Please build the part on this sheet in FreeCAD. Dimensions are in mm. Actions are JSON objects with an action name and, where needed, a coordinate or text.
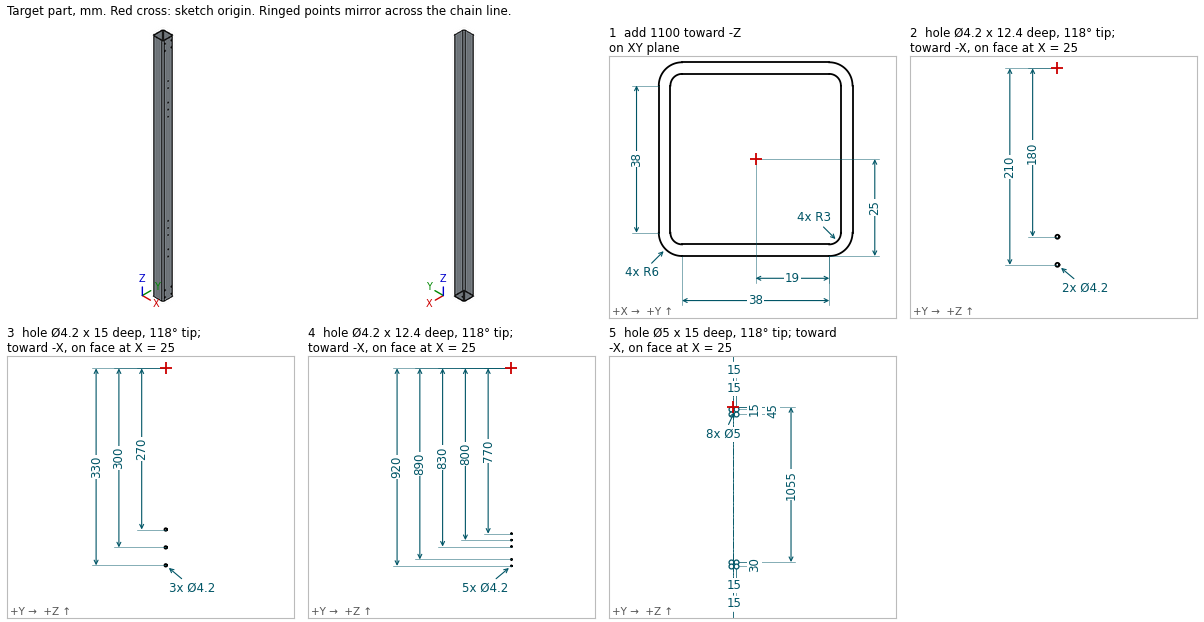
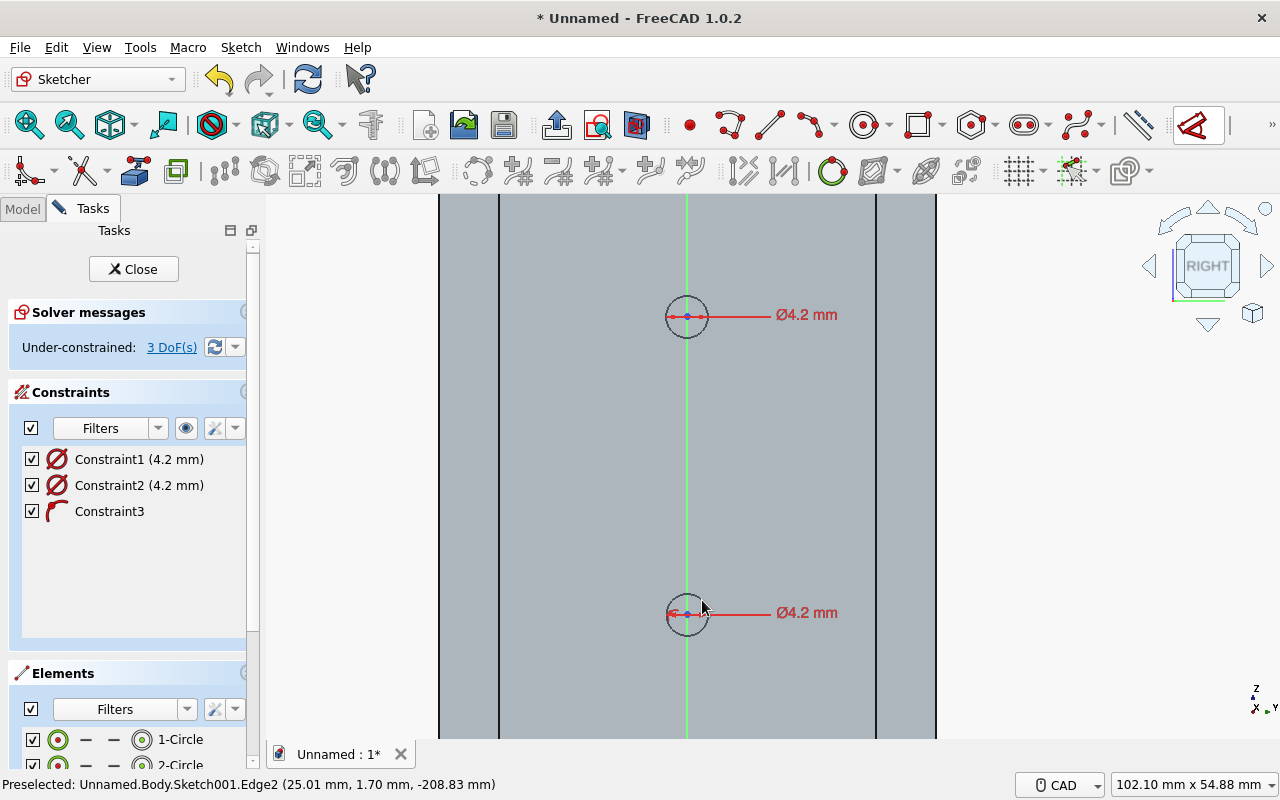
{"action": "left_click", "coordinate": [687, 317]}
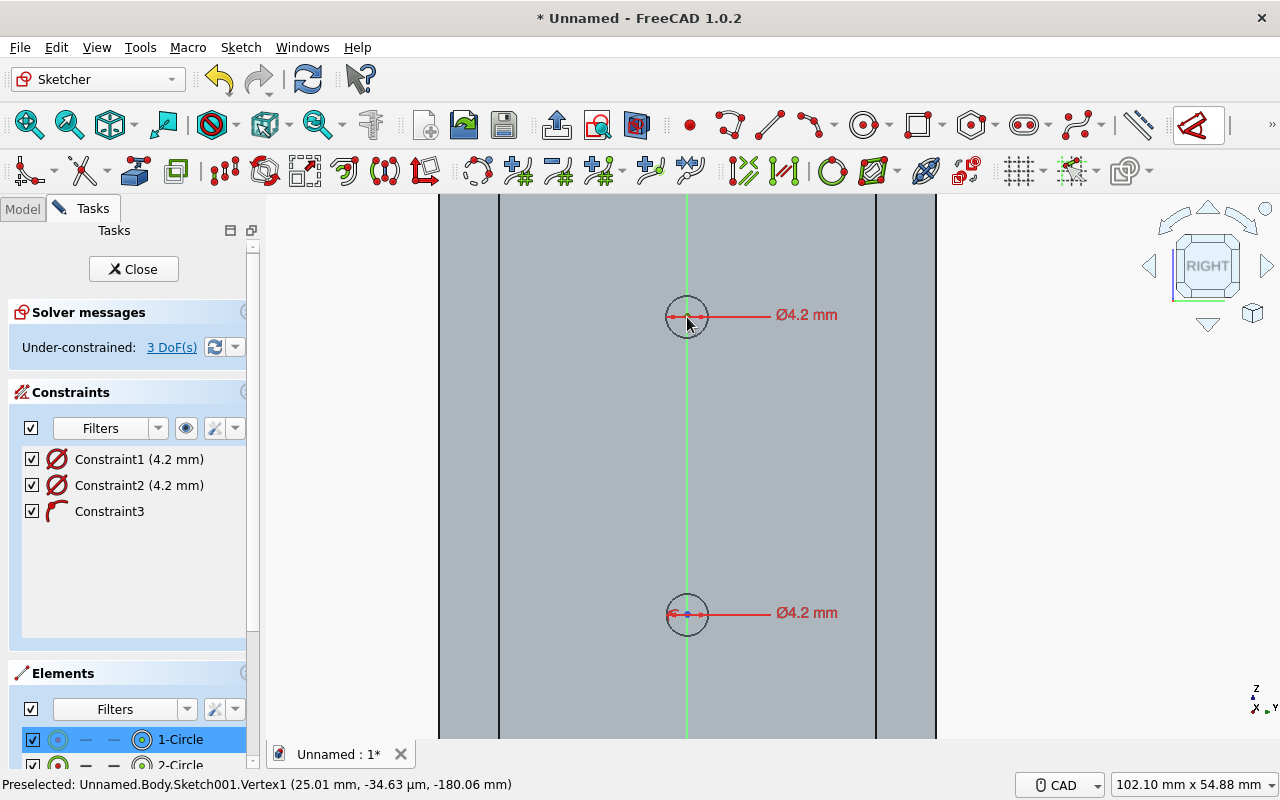
{"action": "left_click", "coordinate": [687, 676]}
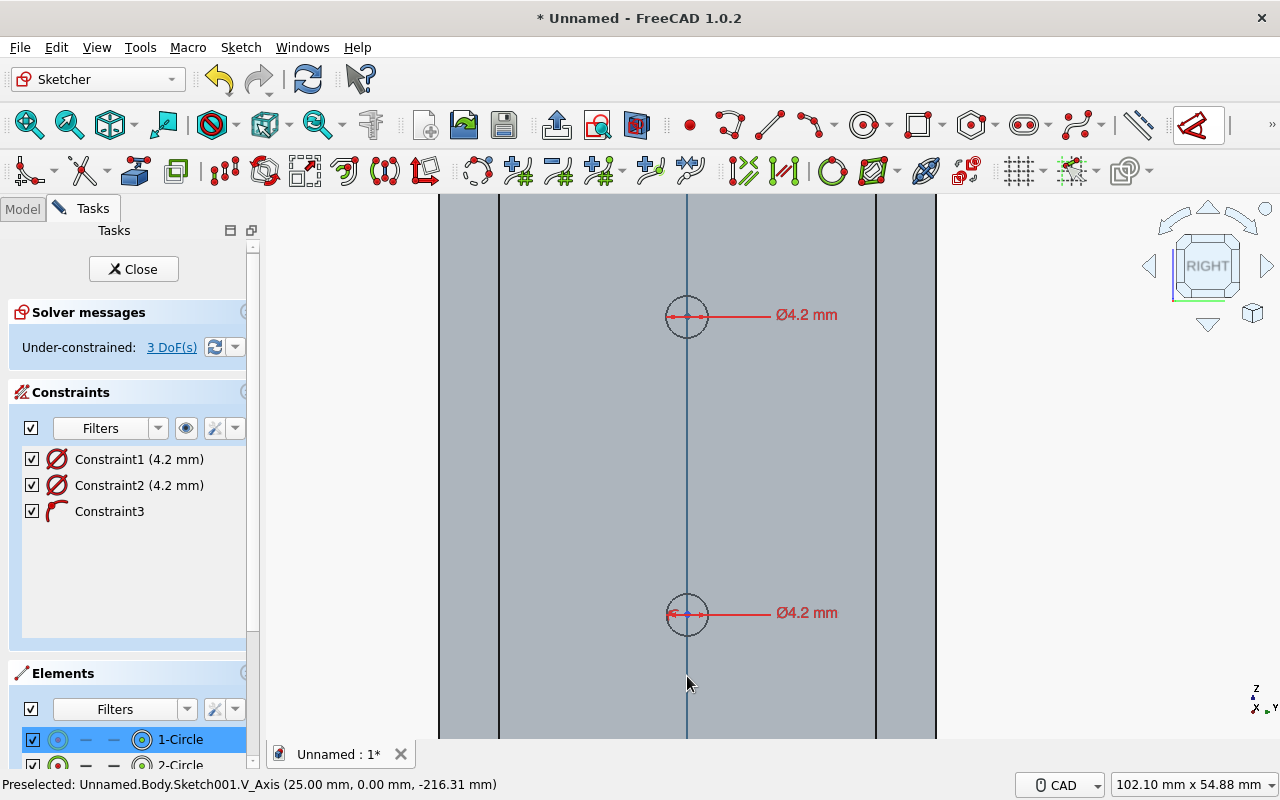
{"action": "key", "text": "c"}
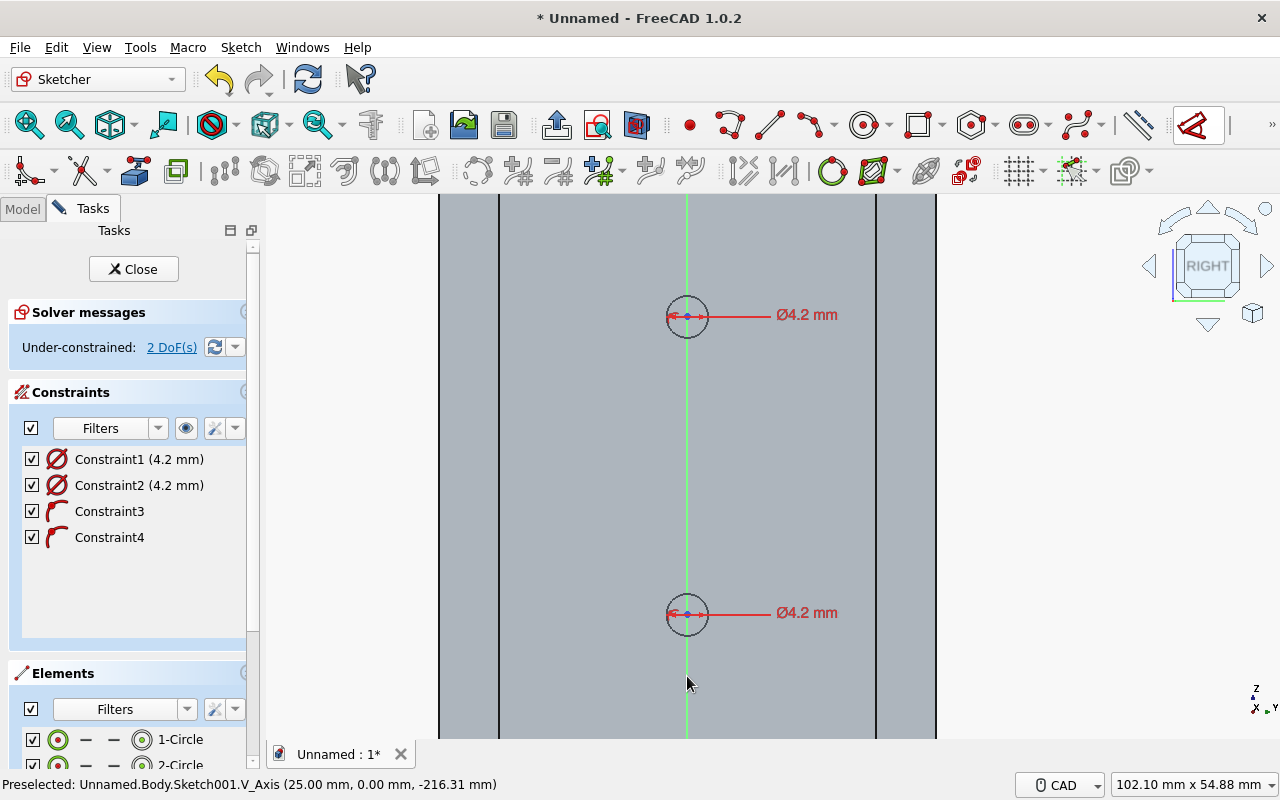
{"action": "left_click", "coordinate": [687, 317]}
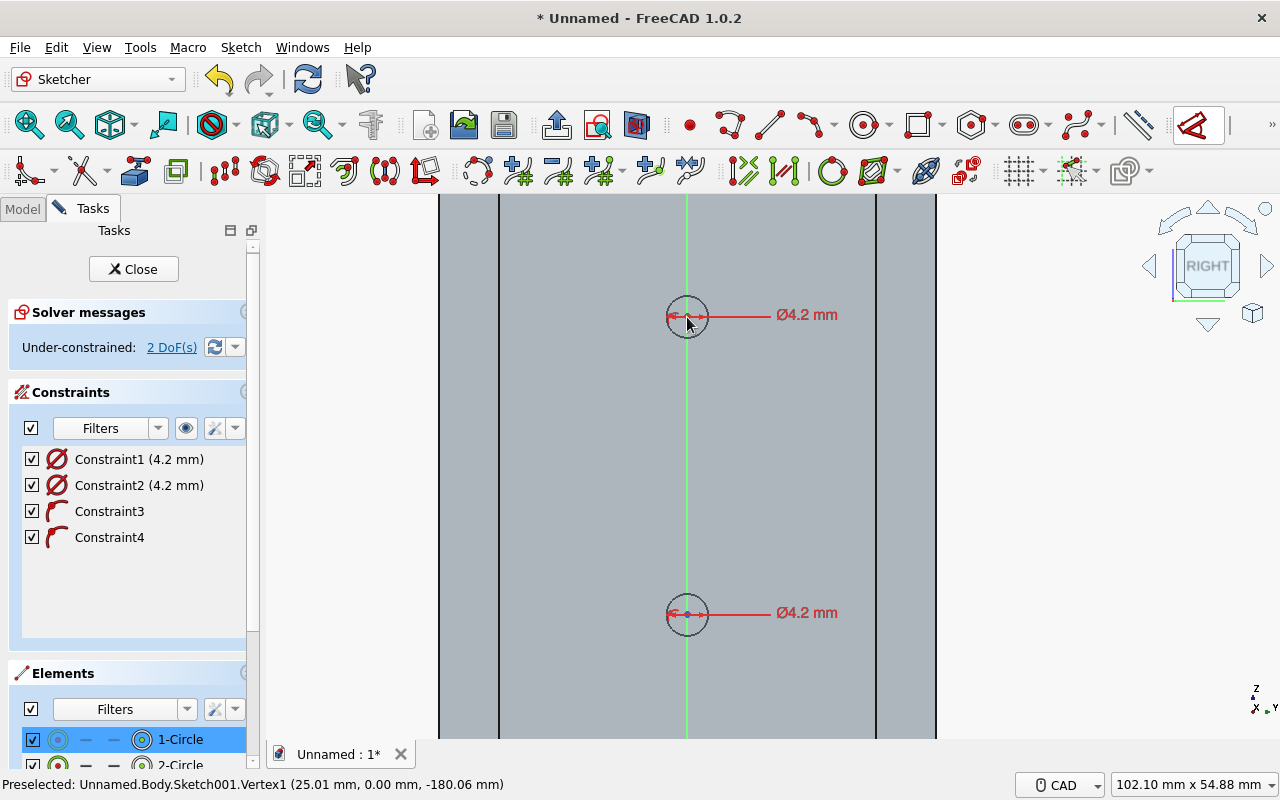
{"action": "left_click", "coordinate": [1218, 126]}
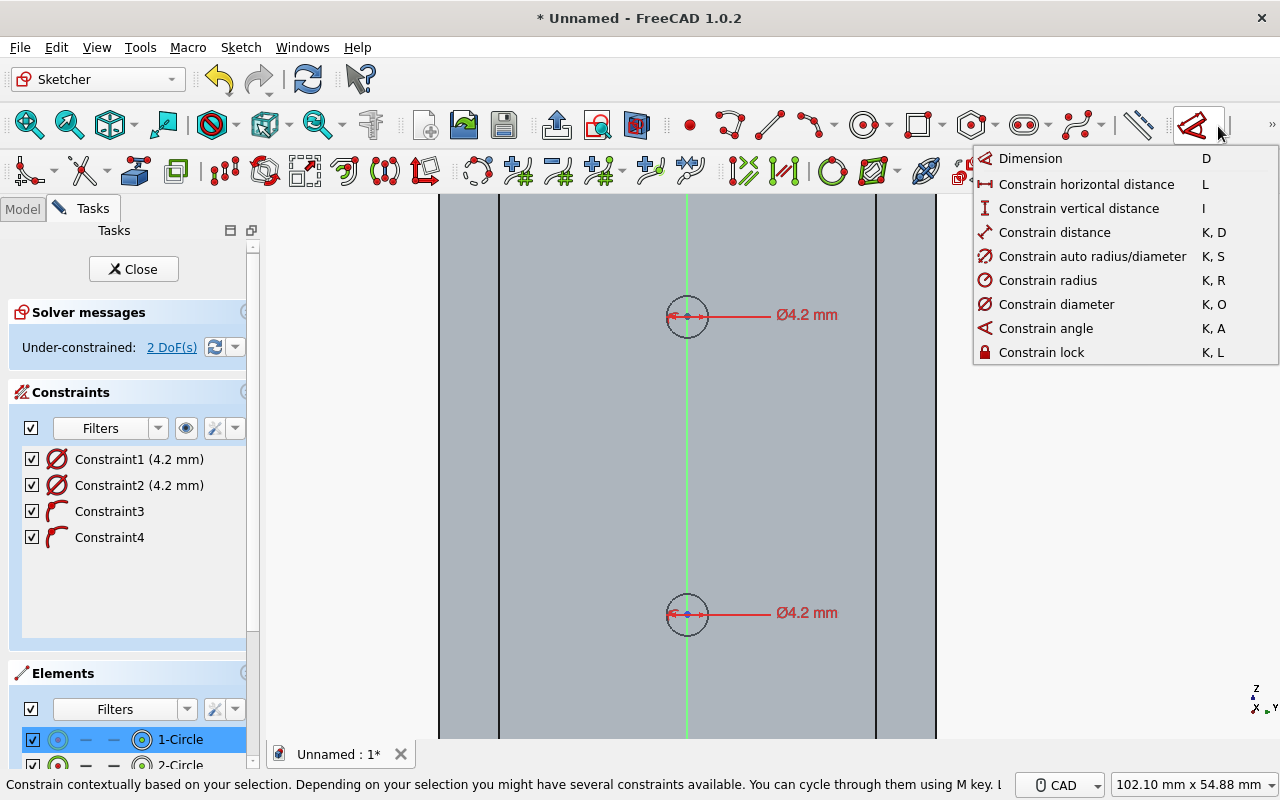
{"action": "left_click", "coordinate": [1126, 208]}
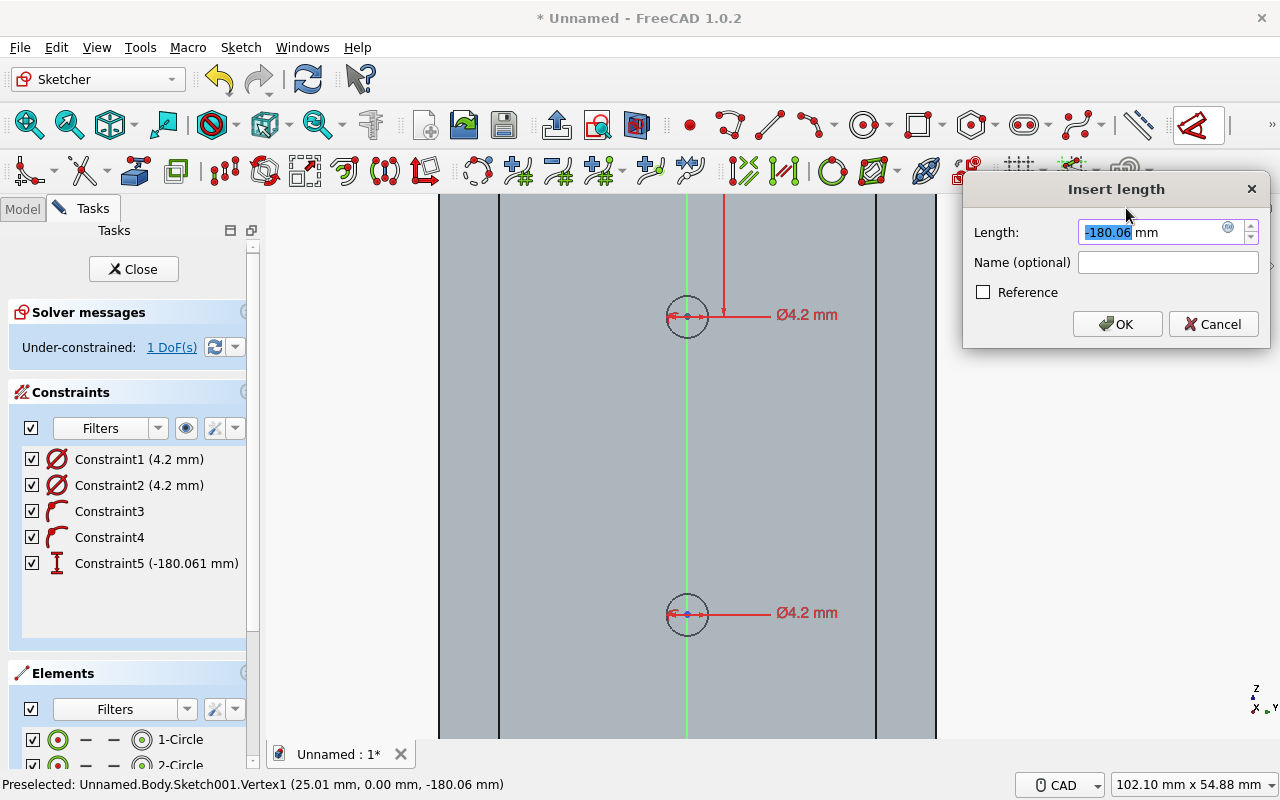
{"action": "type", "text": "-180"}
{"action": "key", "text": "Return"}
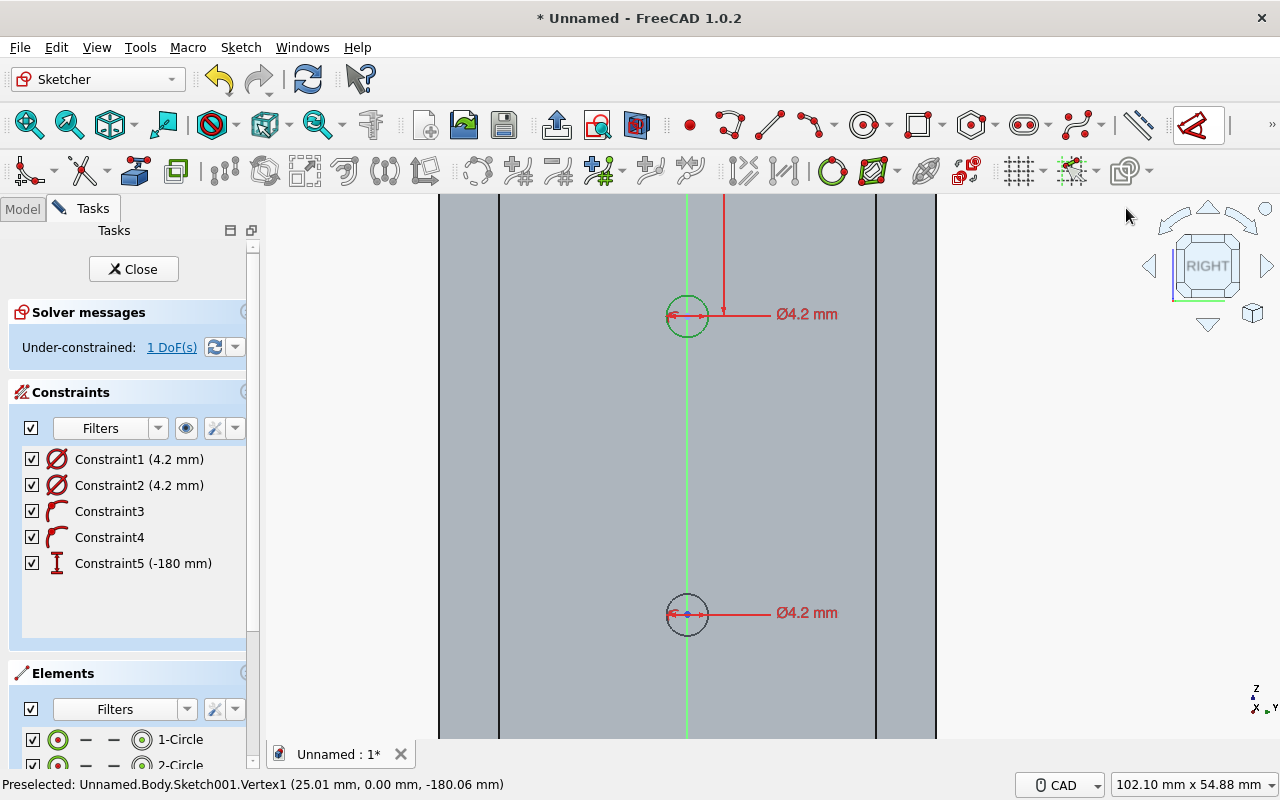
{"action": "left_click", "coordinate": [687, 615]}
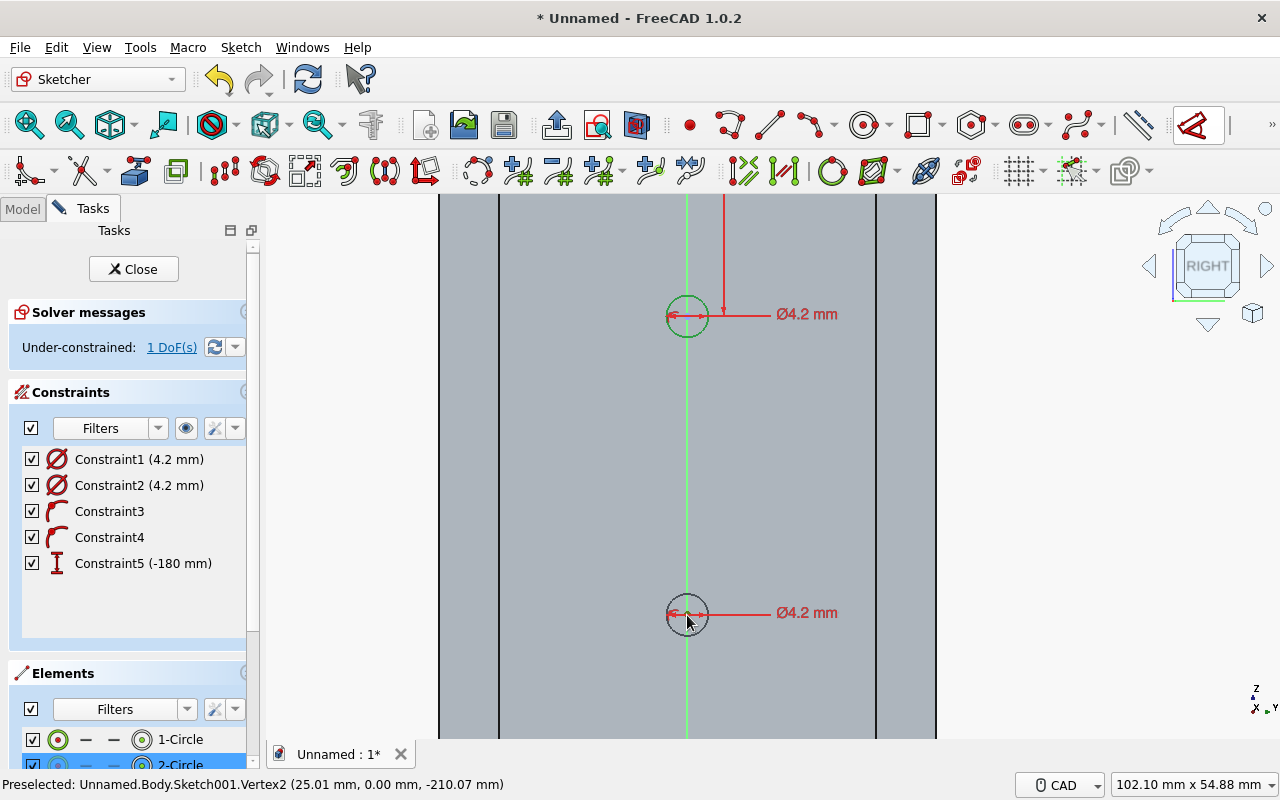
{"action": "left_click", "coordinate": [1218, 126]}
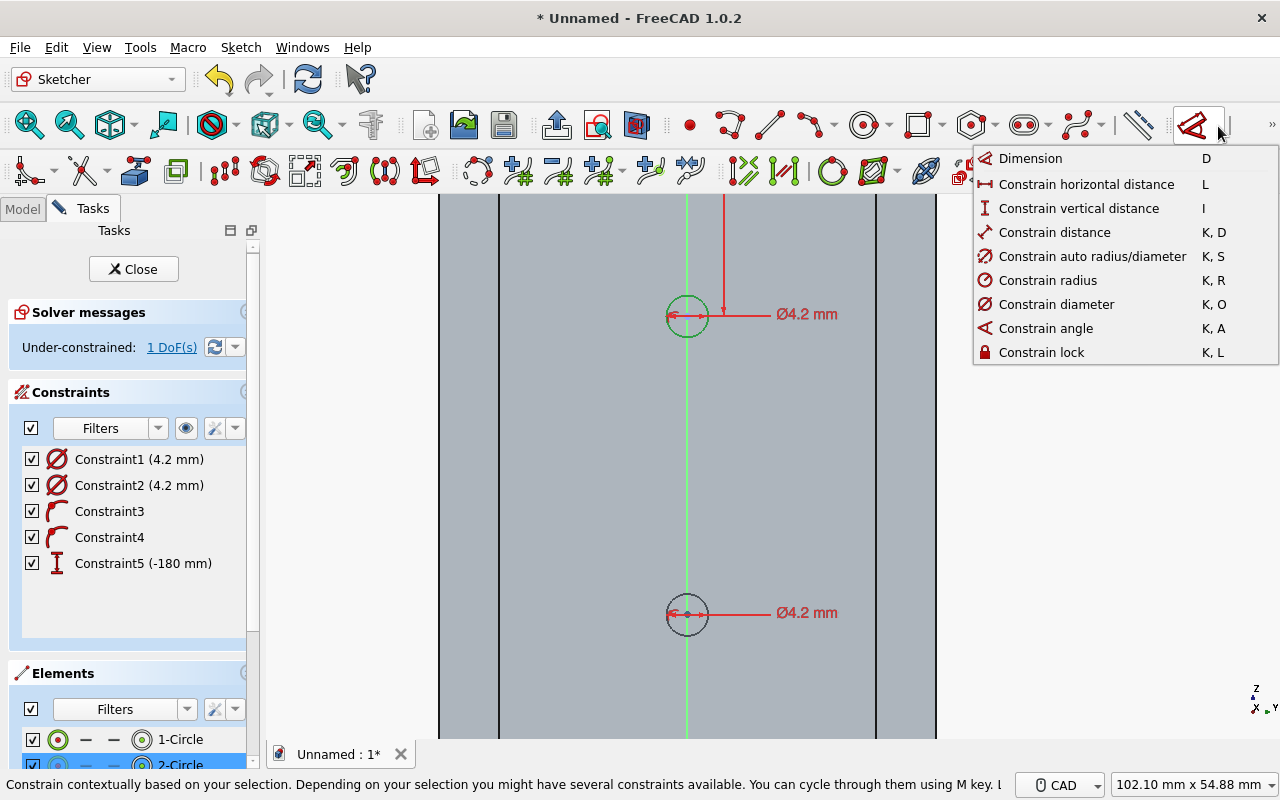
{"action": "left_click", "coordinate": [1126, 208]}